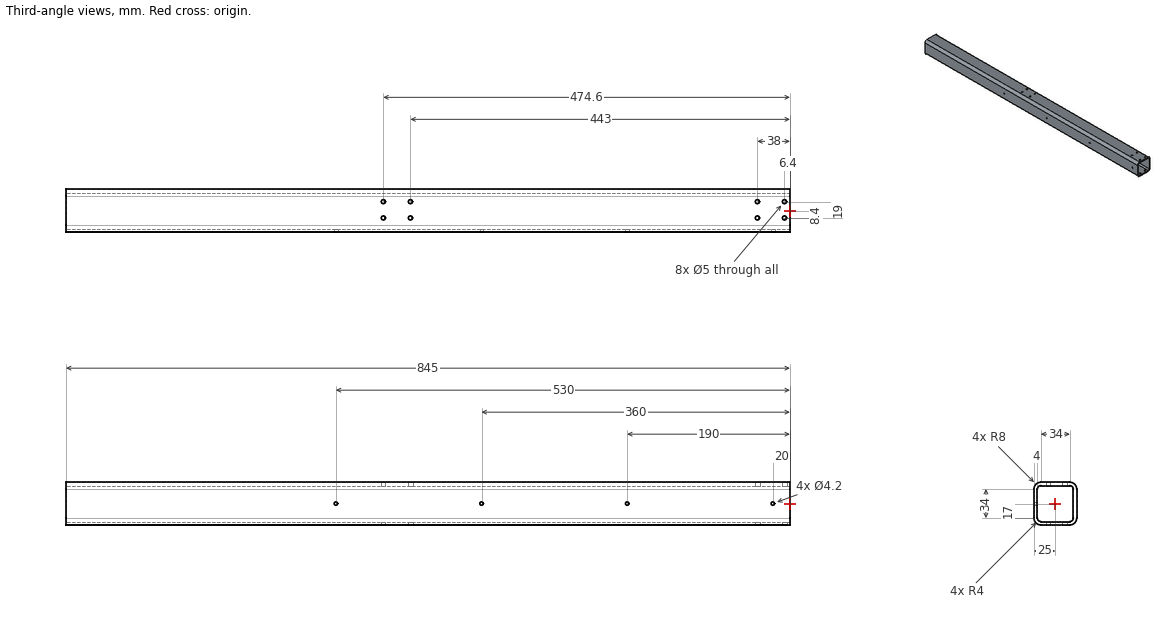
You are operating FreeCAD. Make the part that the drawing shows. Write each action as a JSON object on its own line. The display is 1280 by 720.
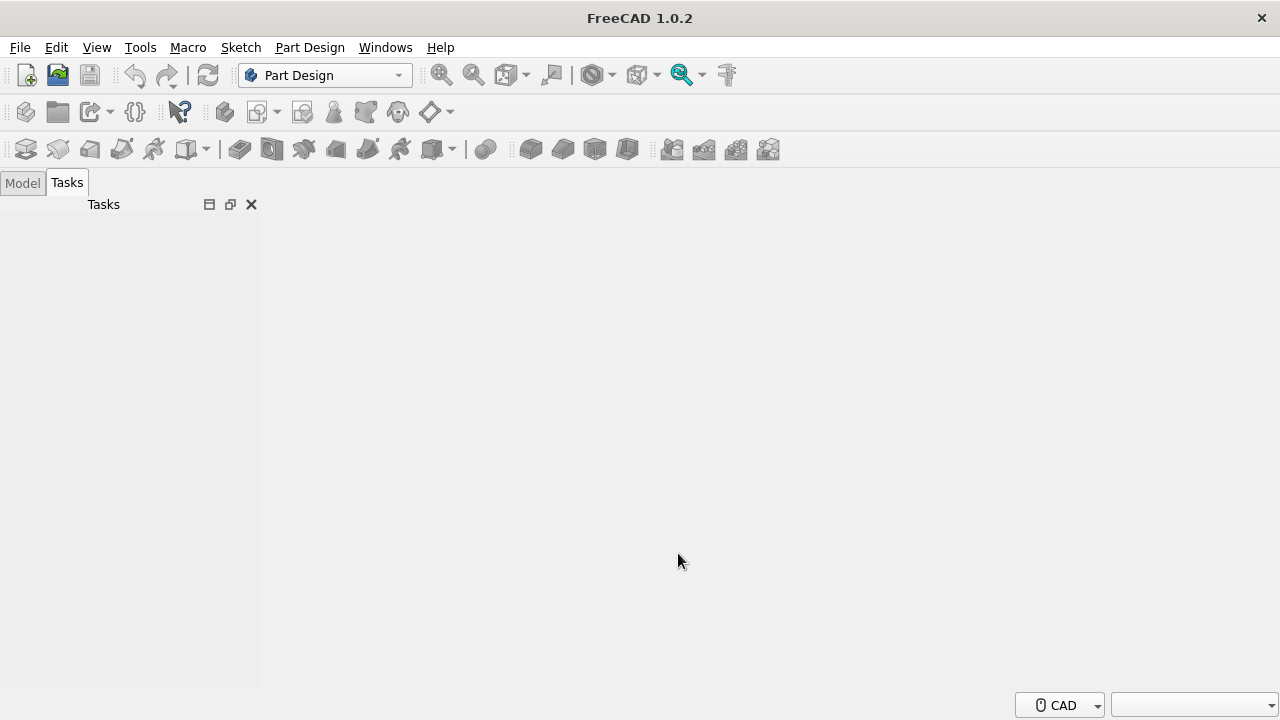
{"action": "left_click", "coordinate": [26, 76]}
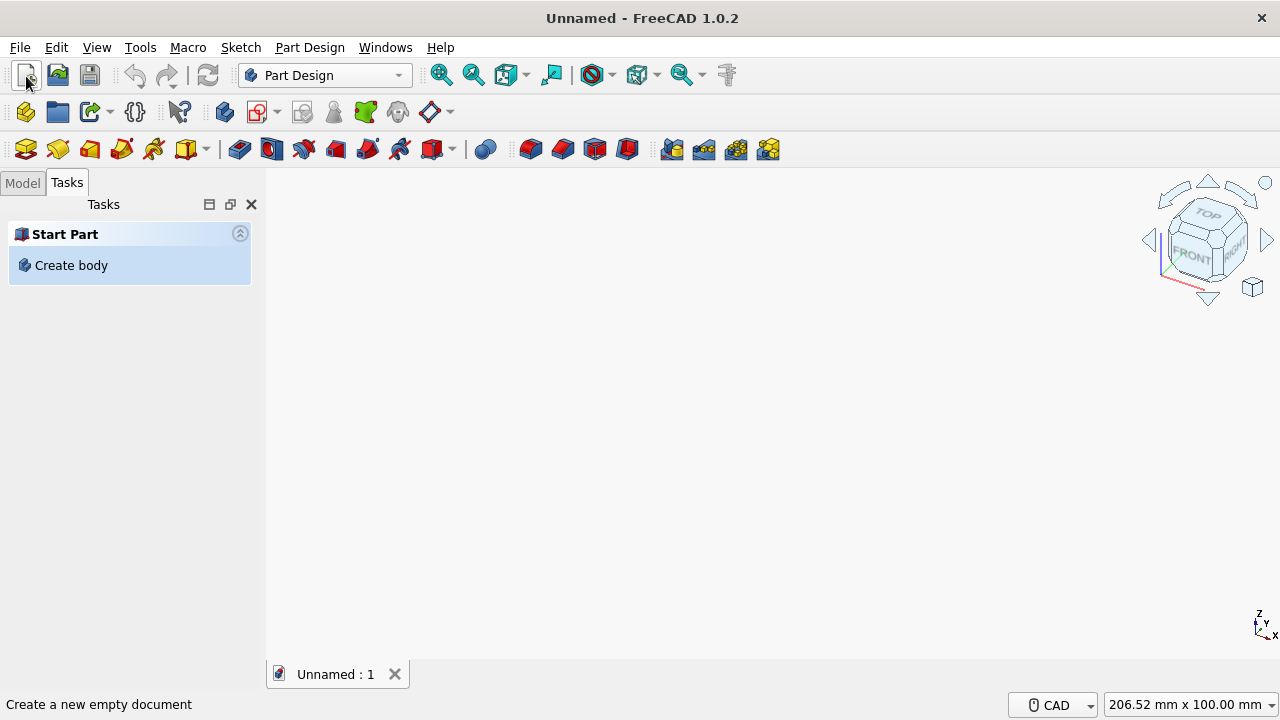
{"action": "left_click", "coordinate": [258, 112]}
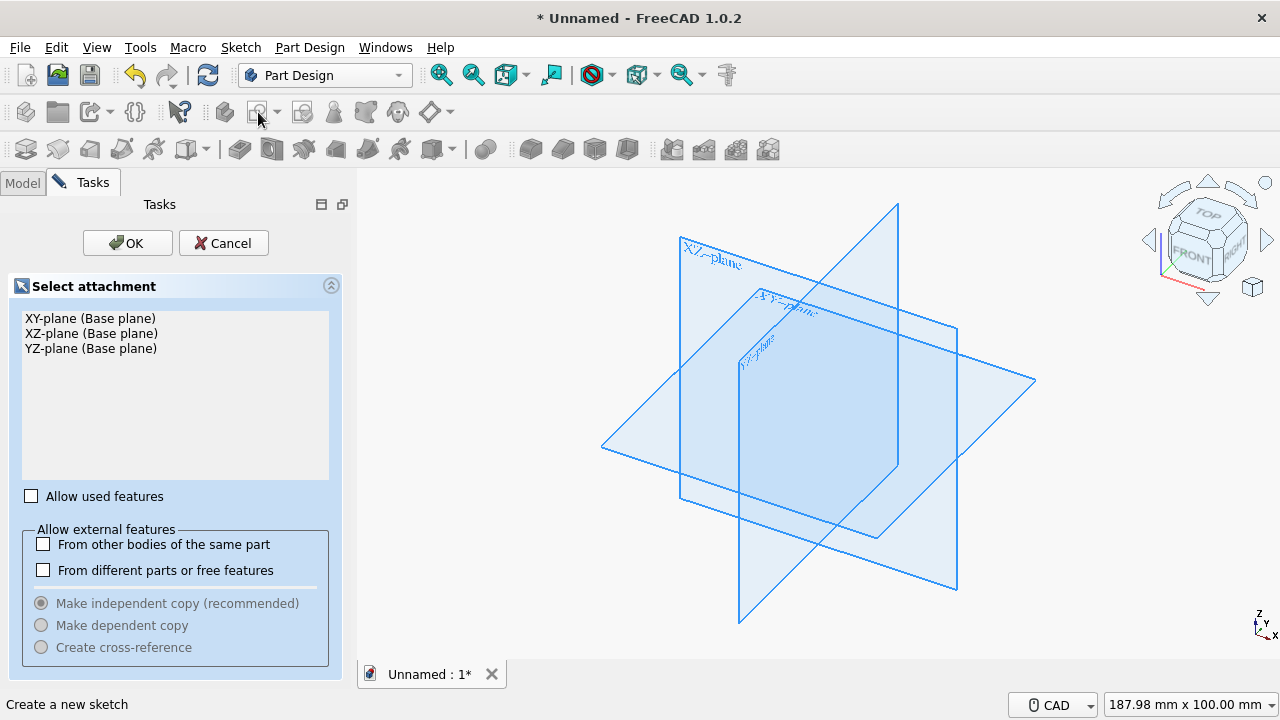
{"action": "left_click", "coordinate": [82, 348]}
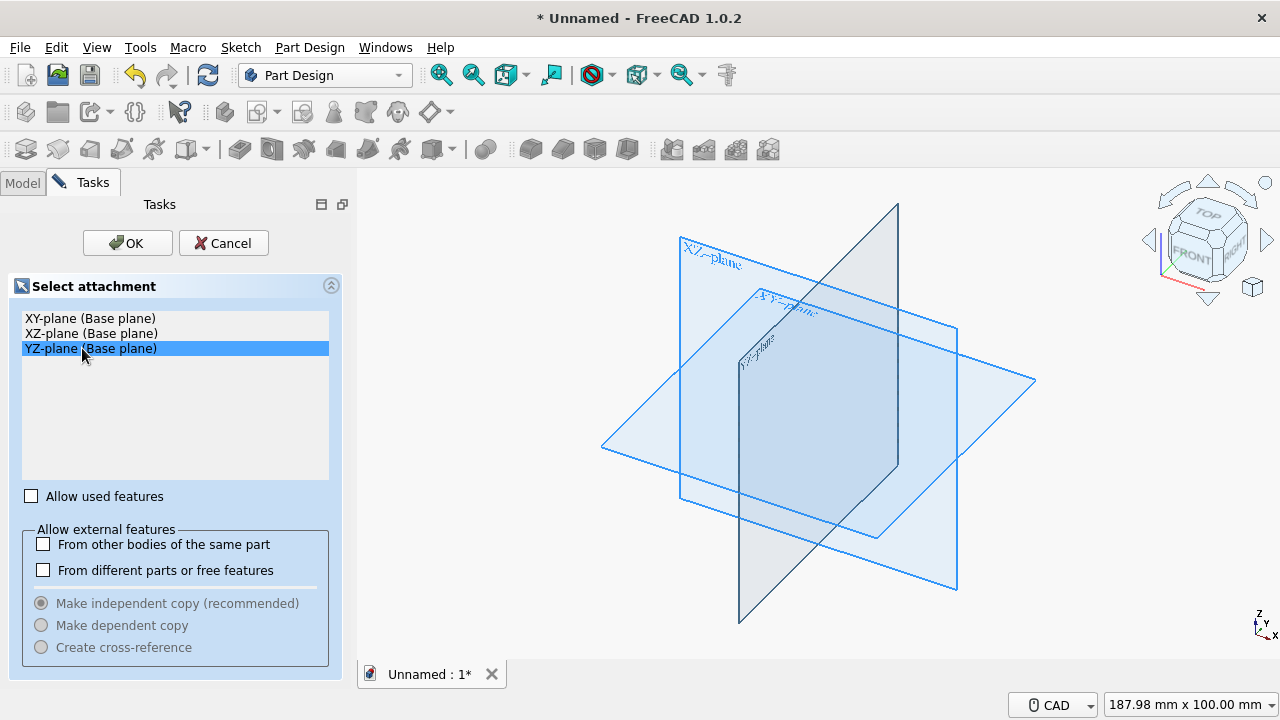
{"action": "left_click", "coordinate": [128, 243]}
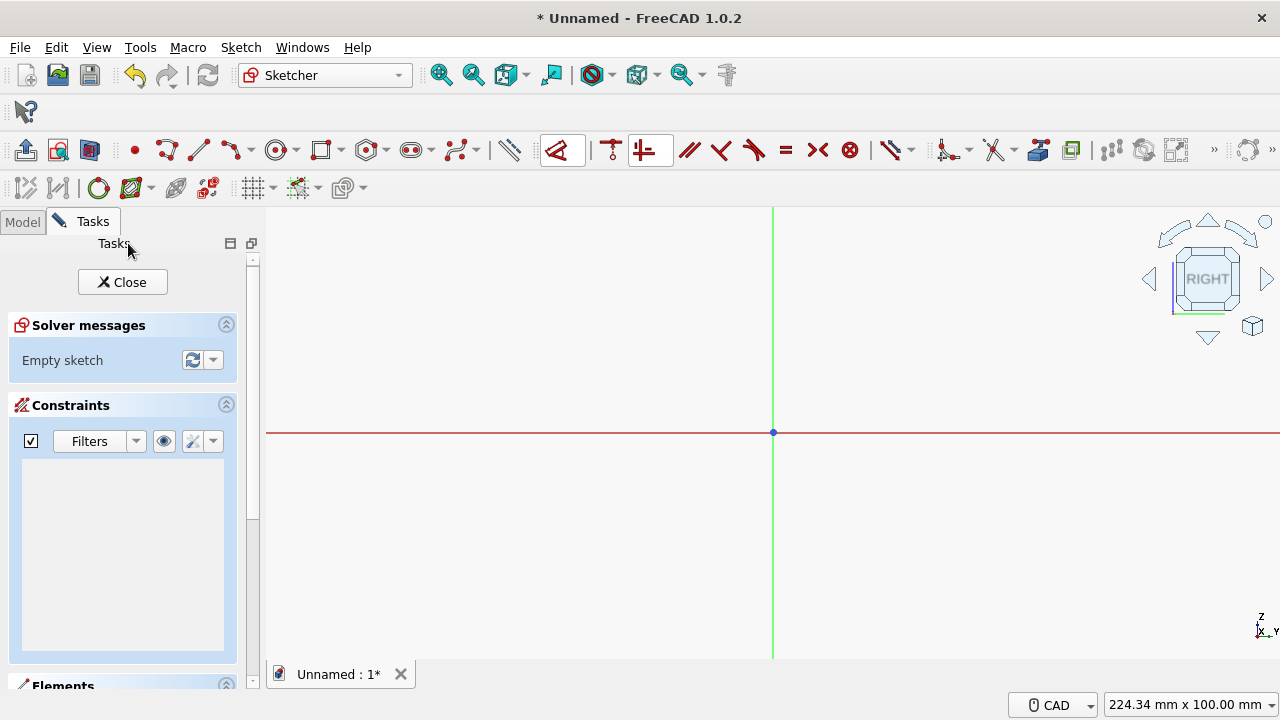
{"action": "left_click", "coordinate": [200, 150]}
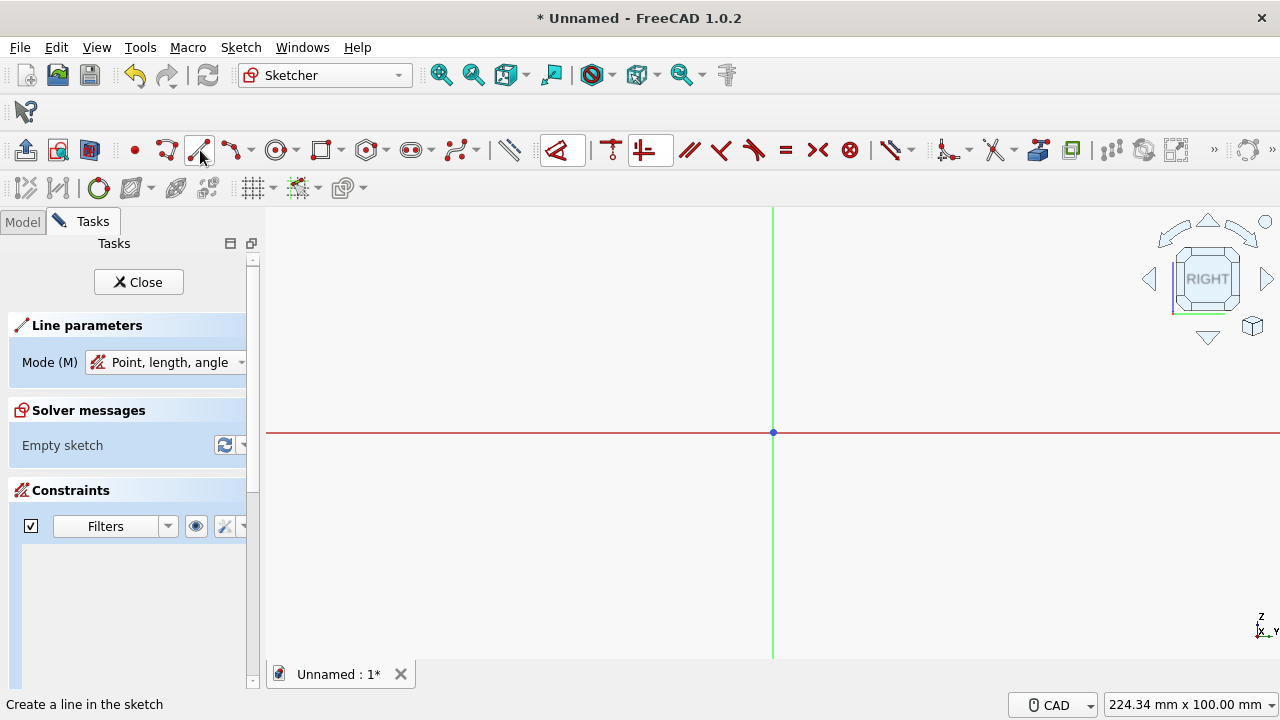
{"action": "left_click", "coordinate": [660, 510]}
{"action": "left_click", "coordinate": [660, 356]}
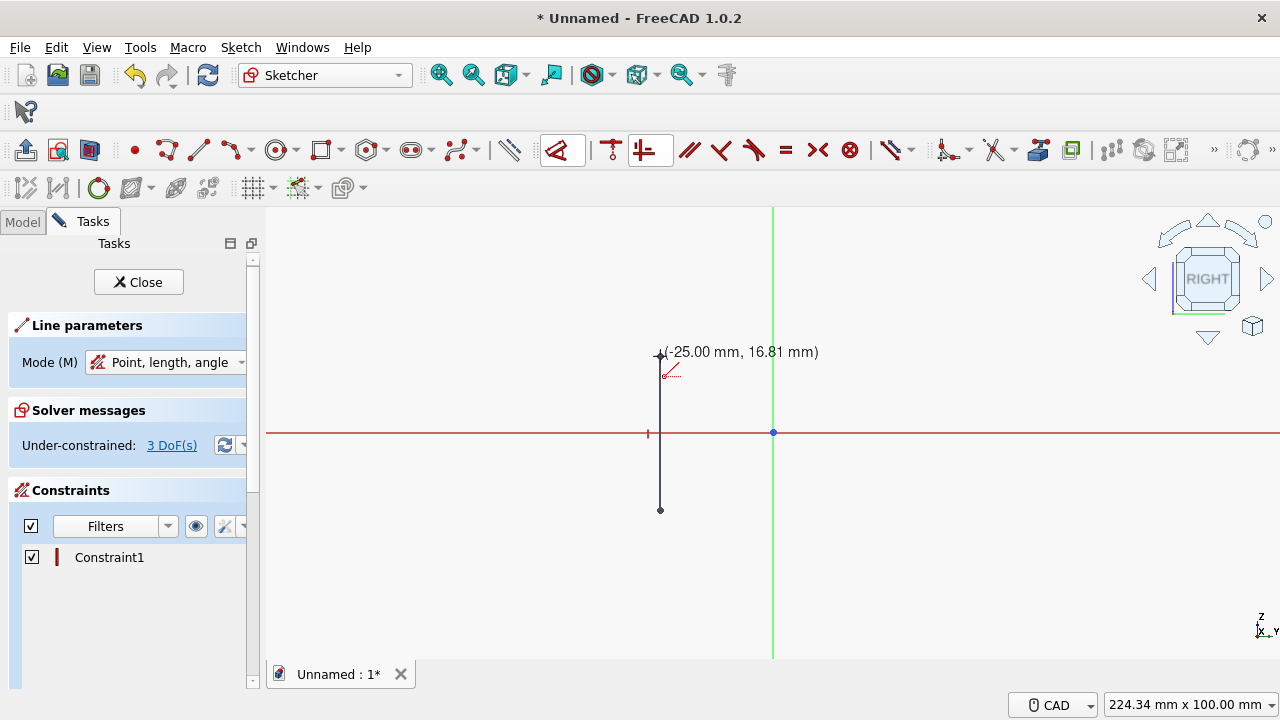
{"action": "left_click", "coordinate": [696, 320]}
{"action": "left_click", "coordinate": [850, 320]}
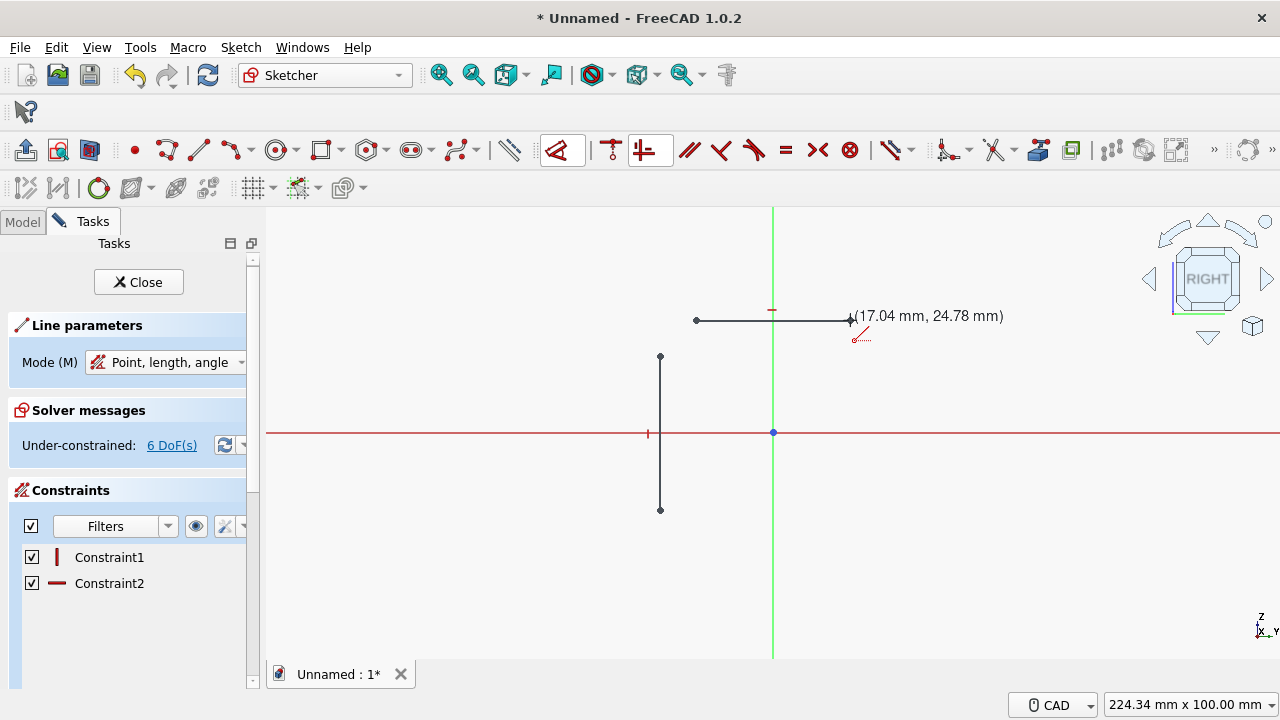
{"action": "left_click", "coordinate": [886, 356]}
{"action": "left_click", "coordinate": [886, 510]}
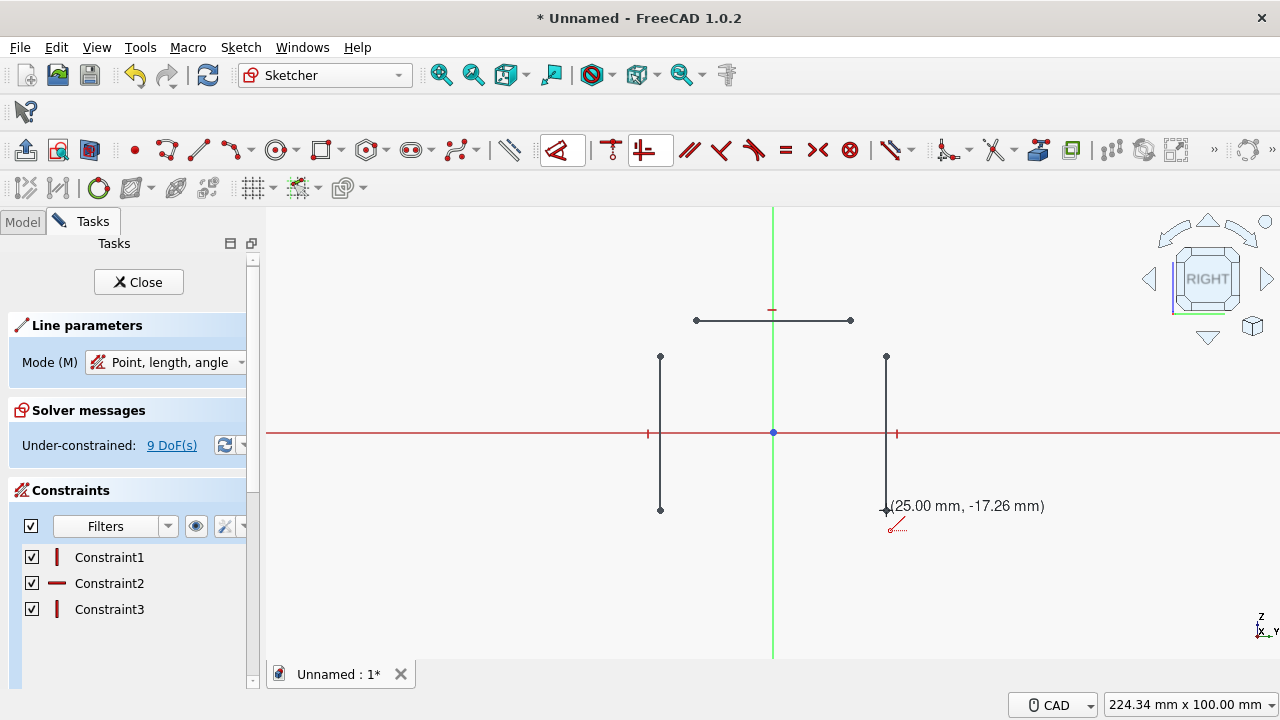
{"action": "left_click", "coordinate": [850, 546]}
{"action": "left_click", "coordinate": [696, 546]}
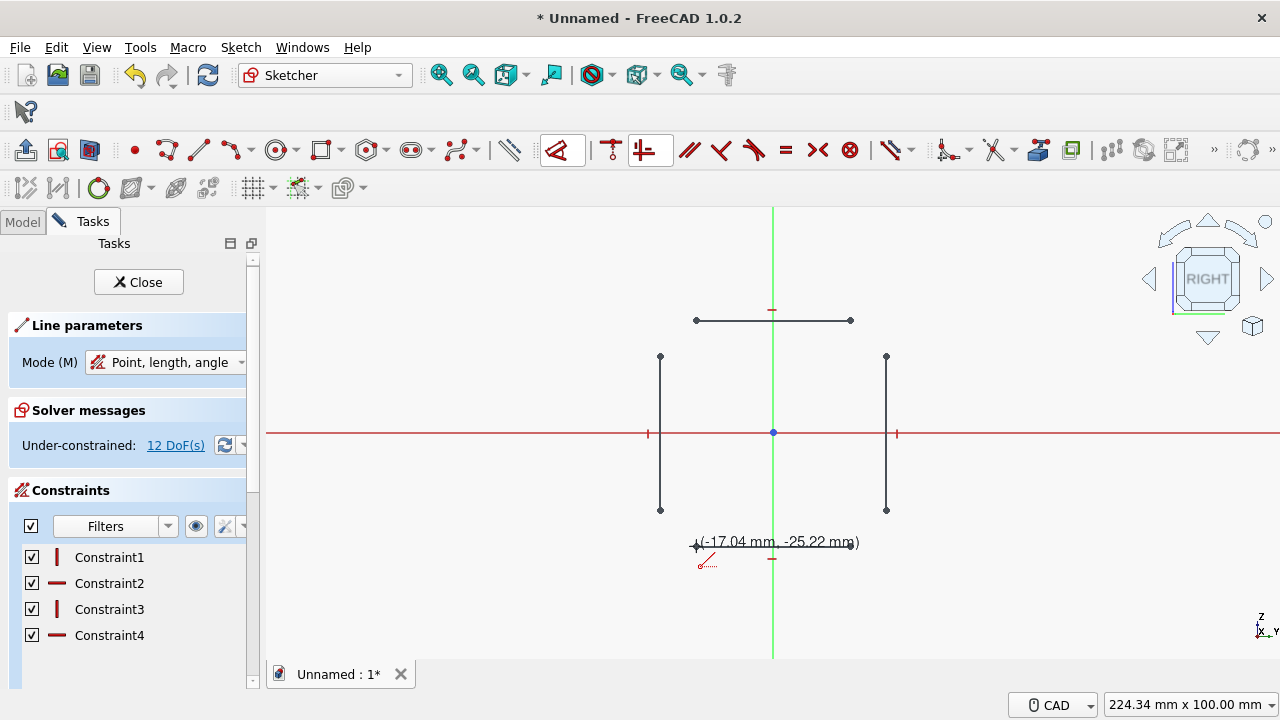
{"action": "left_click", "coordinate": [232, 150]}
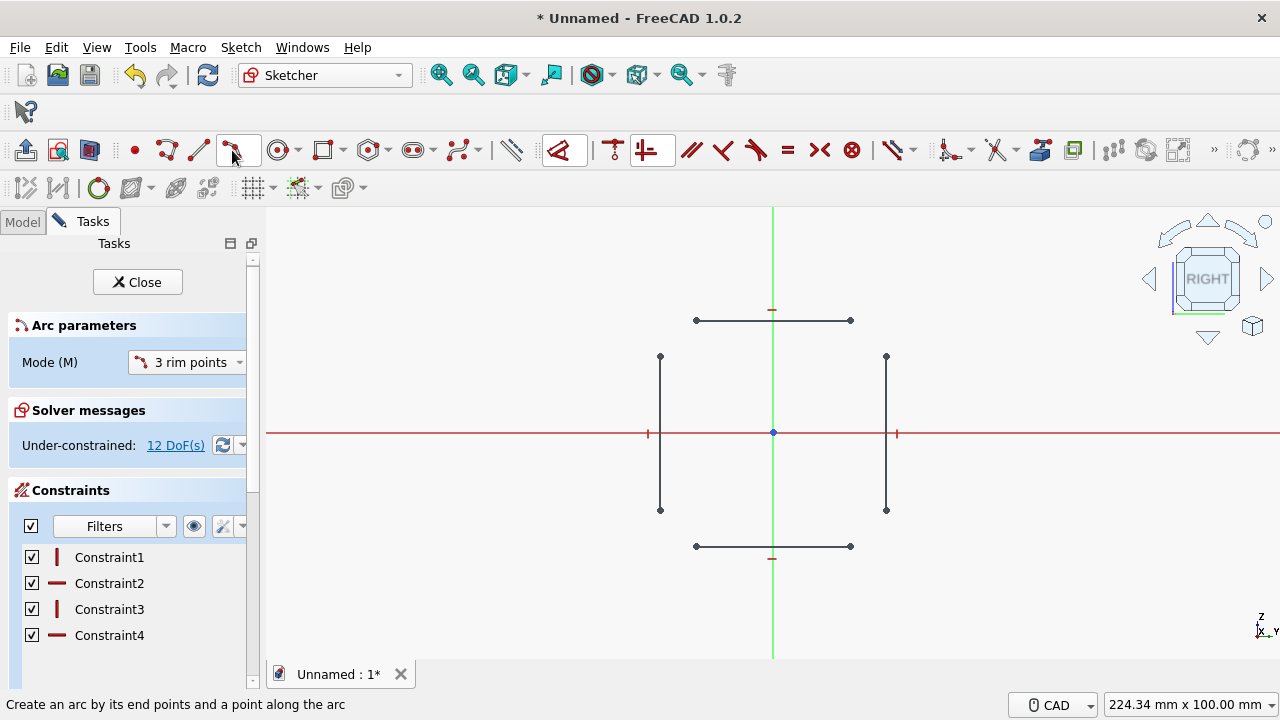
{"action": "left_click", "coordinate": [660, 357]}
{"action": "left_click", "coordinate": [696, 321]}